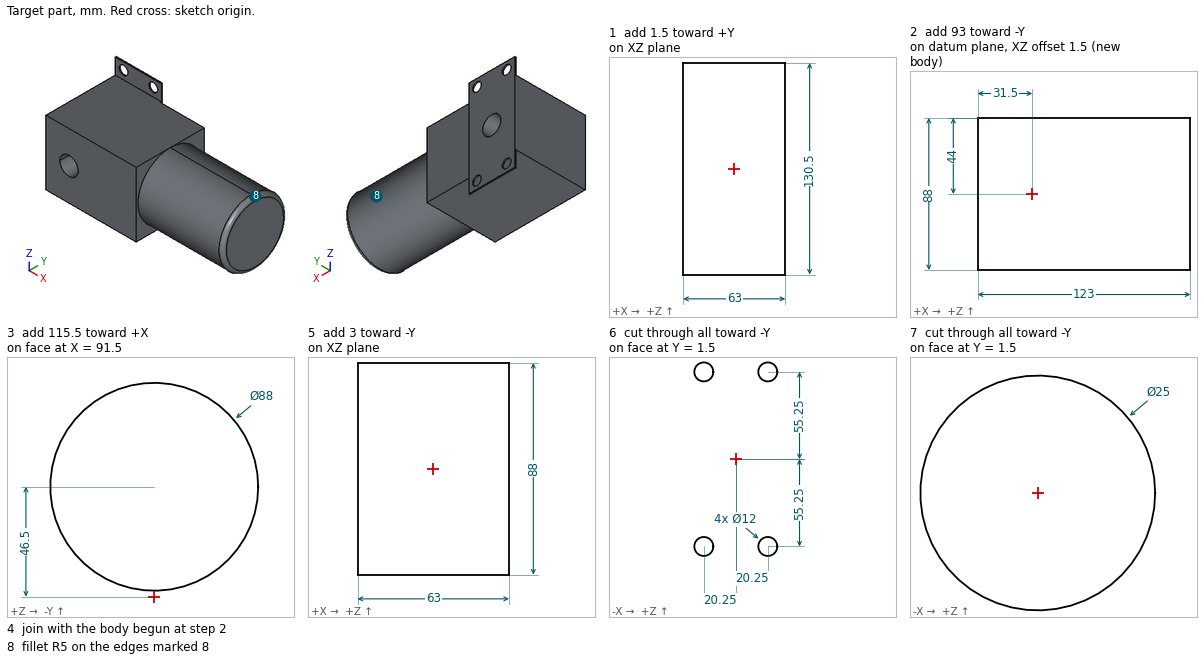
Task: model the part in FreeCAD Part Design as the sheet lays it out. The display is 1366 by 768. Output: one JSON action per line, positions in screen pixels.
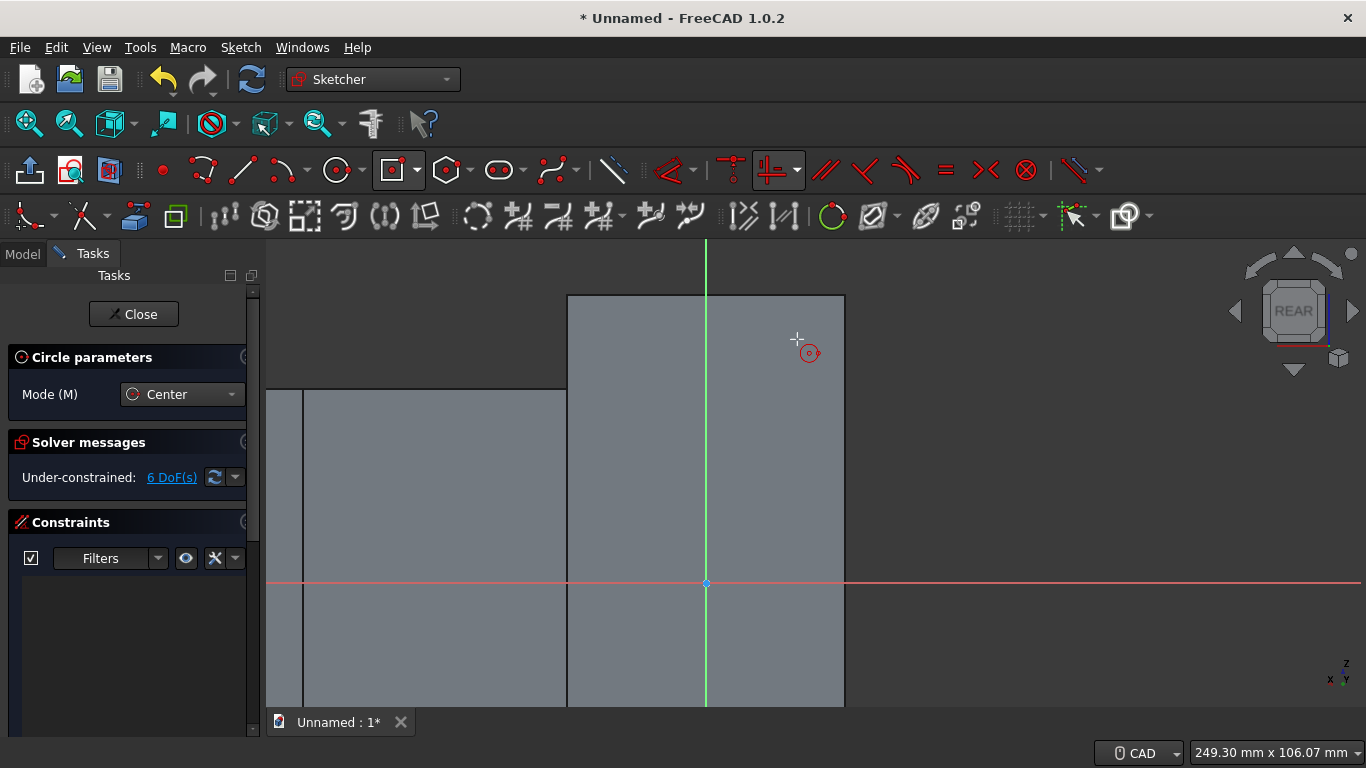
{"action": "left_click", "coordinate": [796, 340]}
{"action": "left_click", "coordinate": [814, 321]}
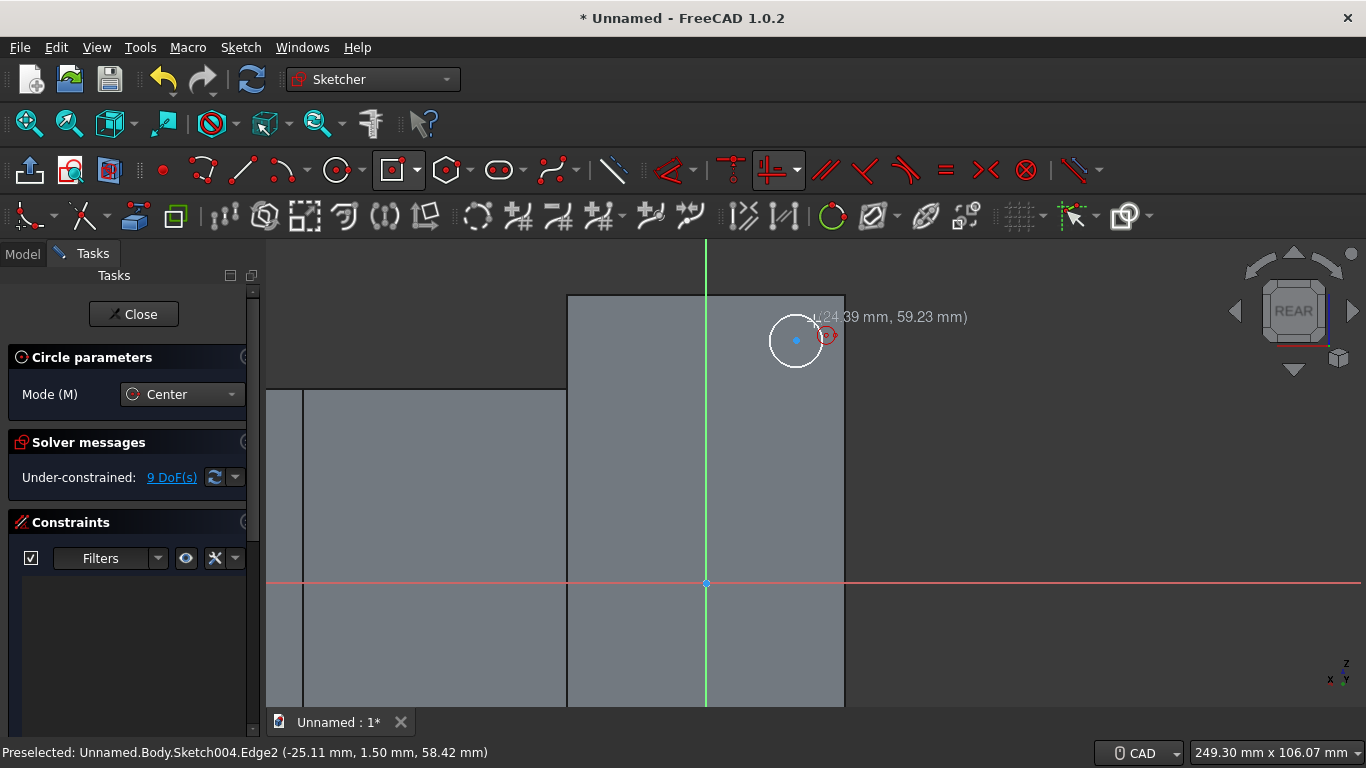
{"action": "left_click", "coordinate": [617, 340]}
{"action": "left_click", "coordinate": [636, 321]}
{"action": "key", "text": "Escape"}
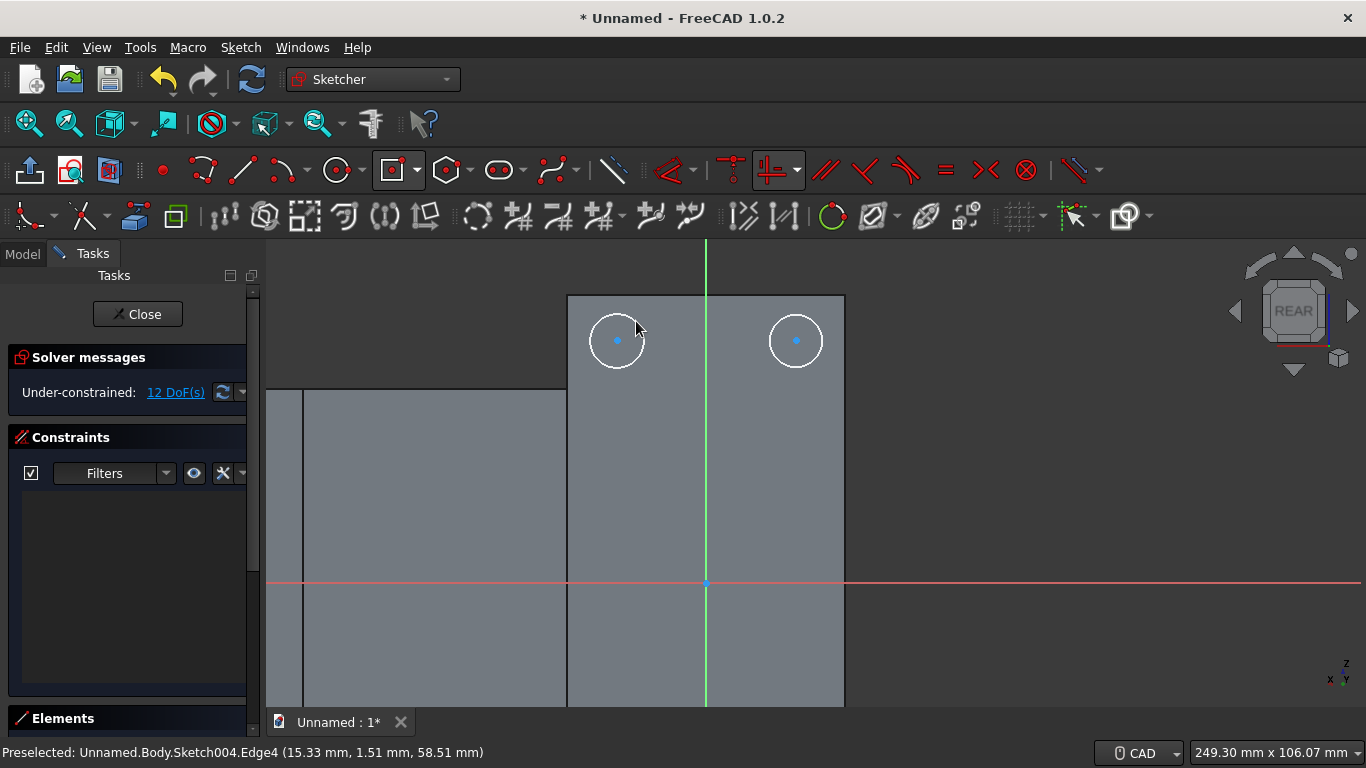
{"action": "scroll", "coordinate": [797, 339], "scroll_direction": "down", "scroll_amount": 3}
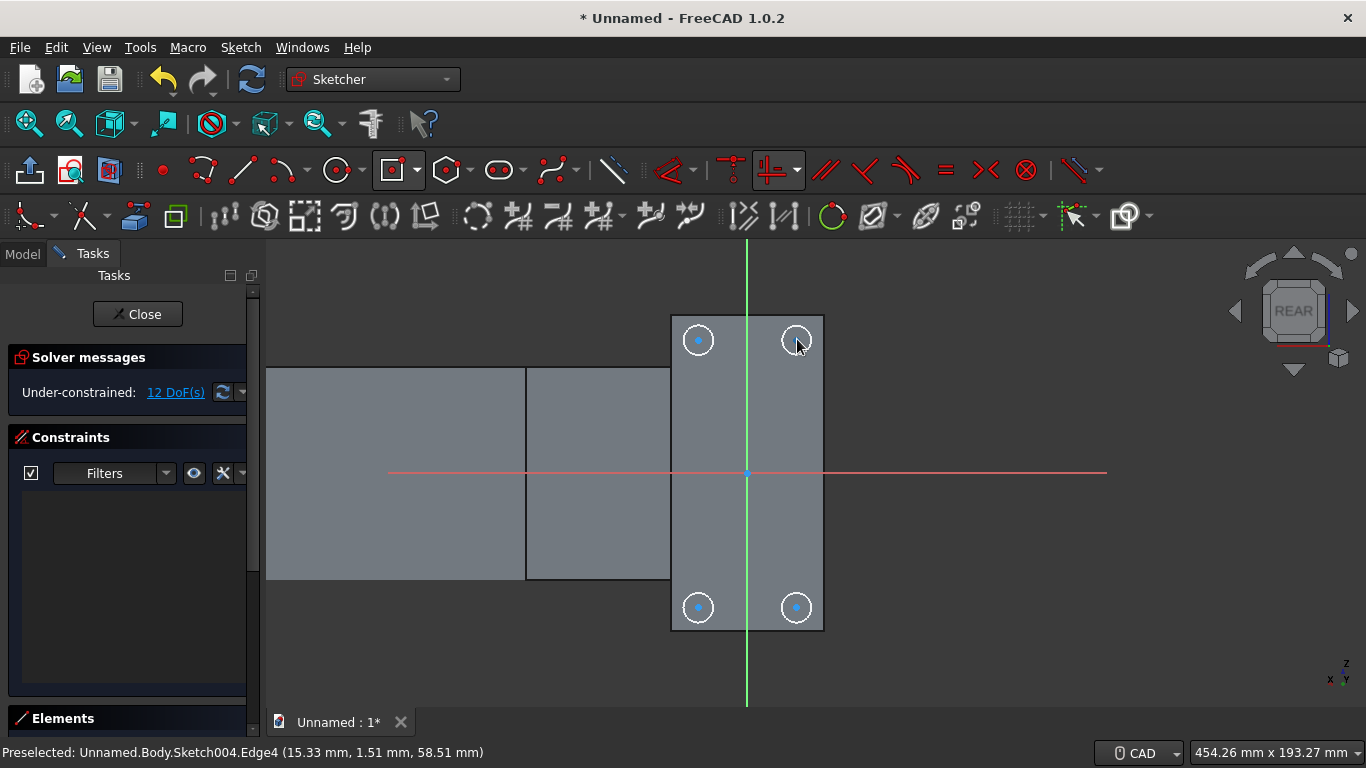
{"action": "left_click", "coordinate": [807, 597]}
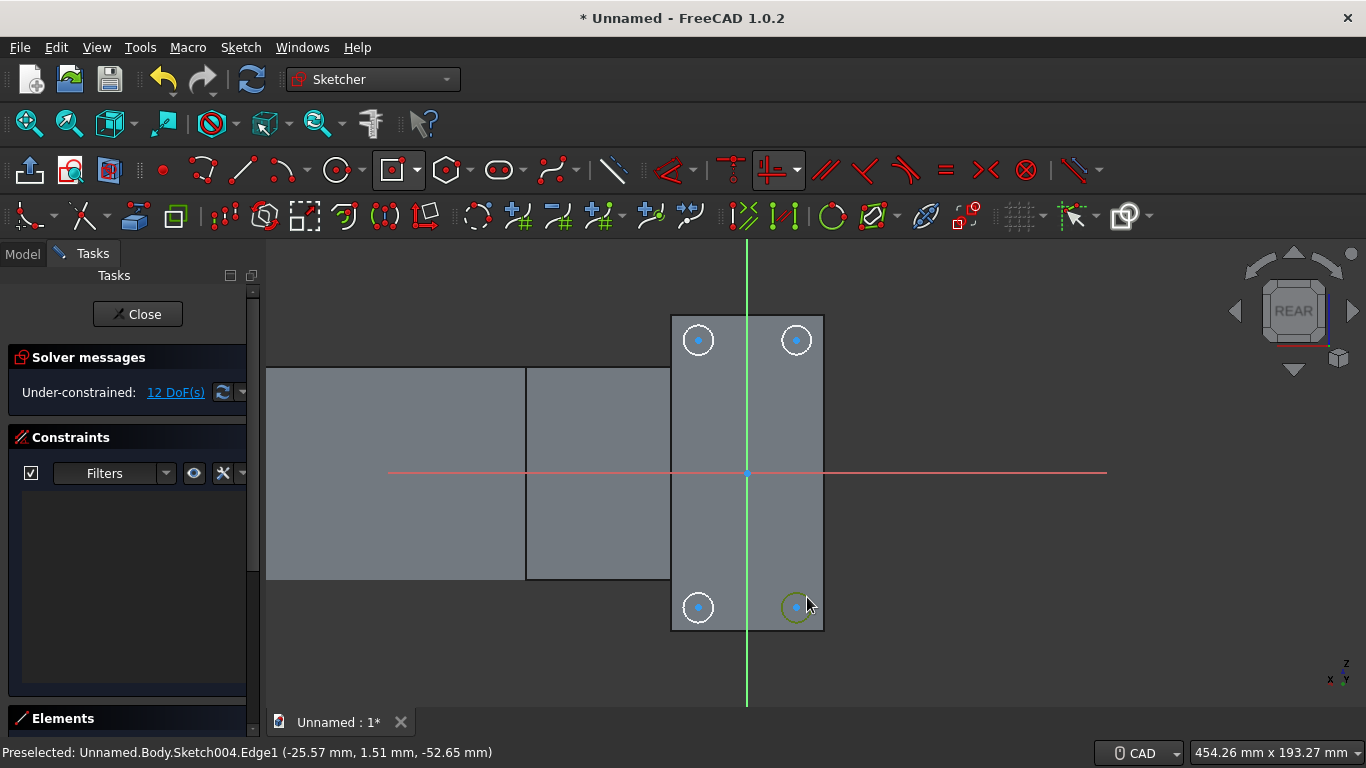
{"action": "left_click", "coordinate": [709, 597]}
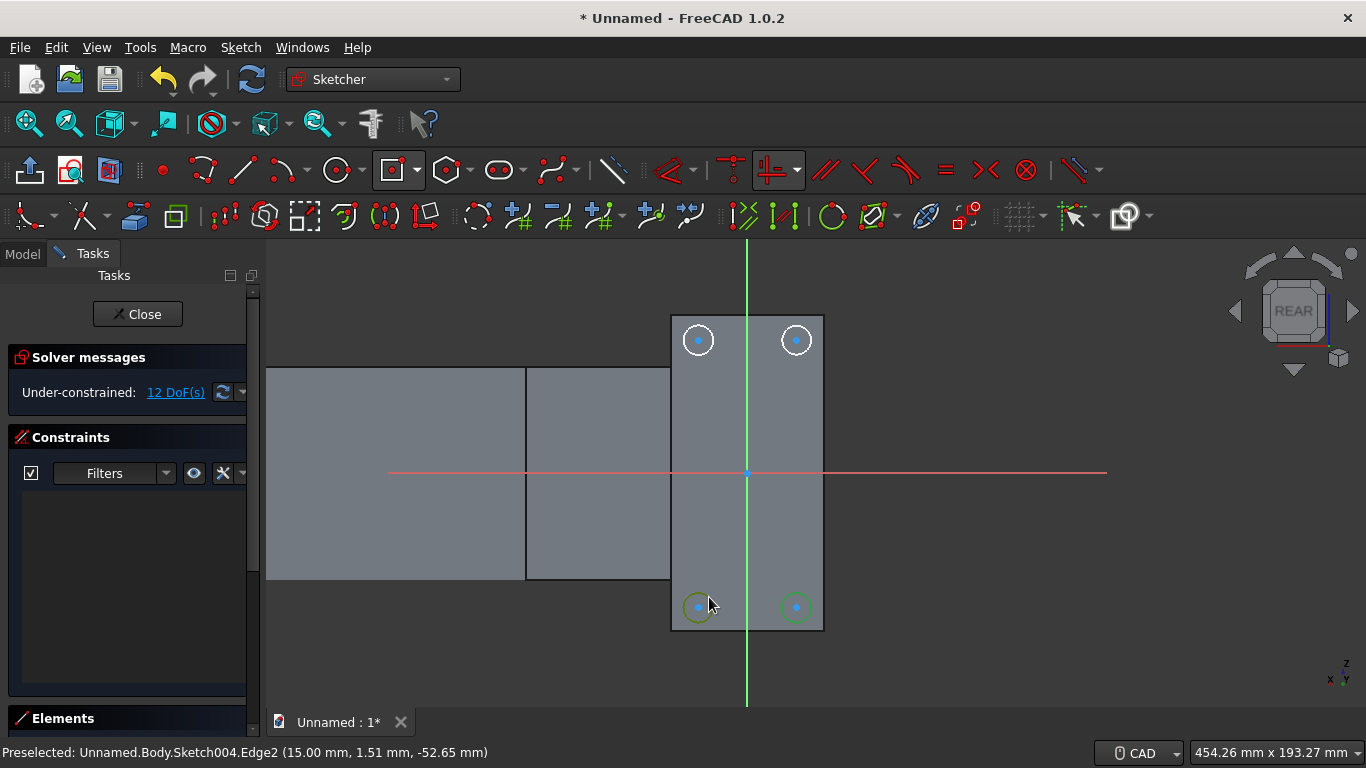
{"action": "left_click", "coordinate": [807, 330]}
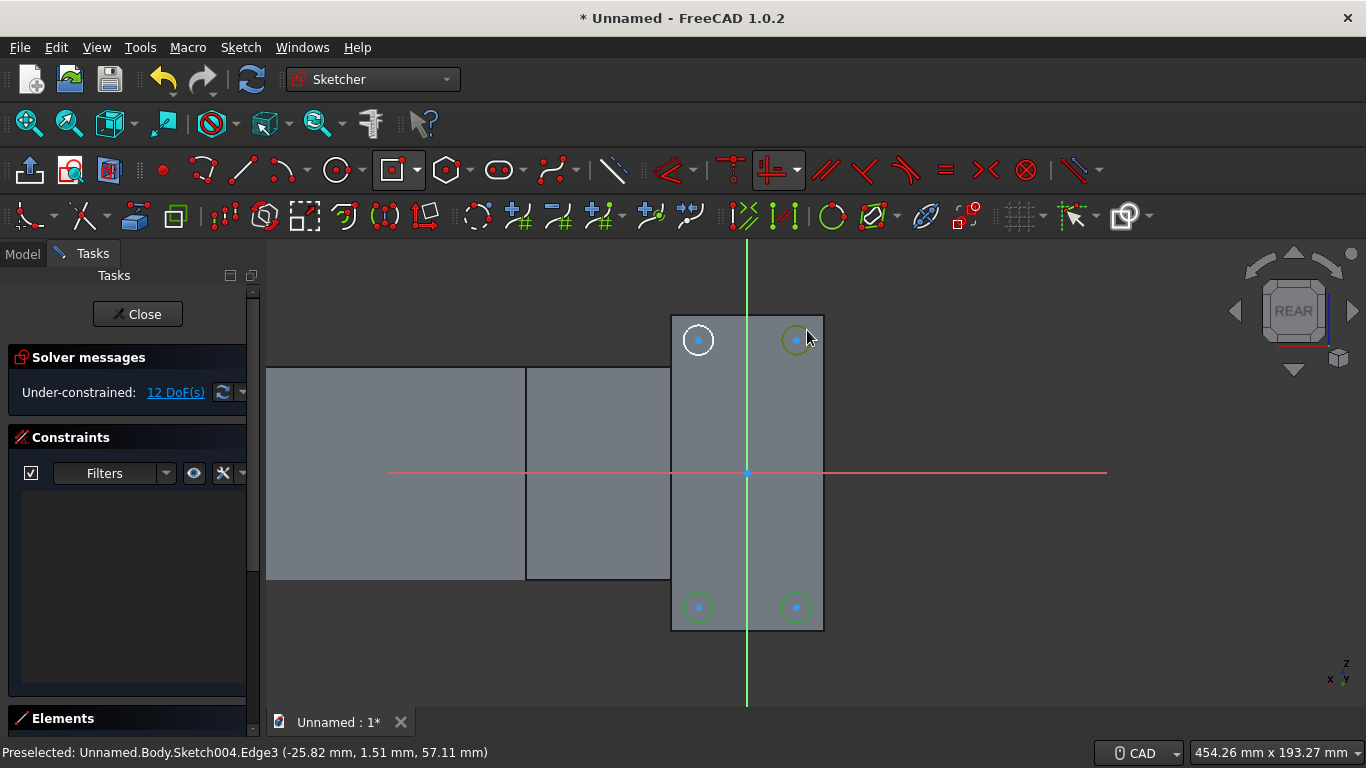
{"action": "left_click", "coordinate": [709, 330]}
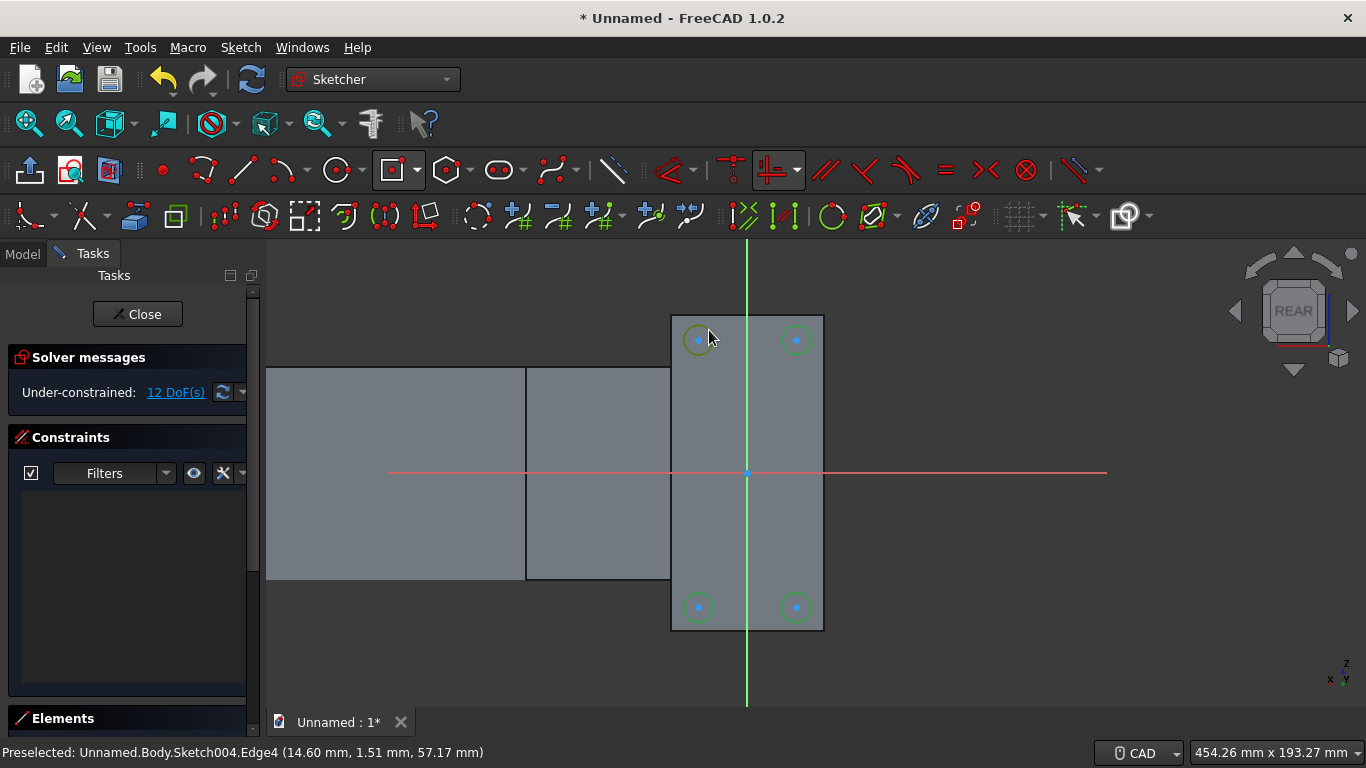
{"action": "left_click", "coordinate": [946, 170]}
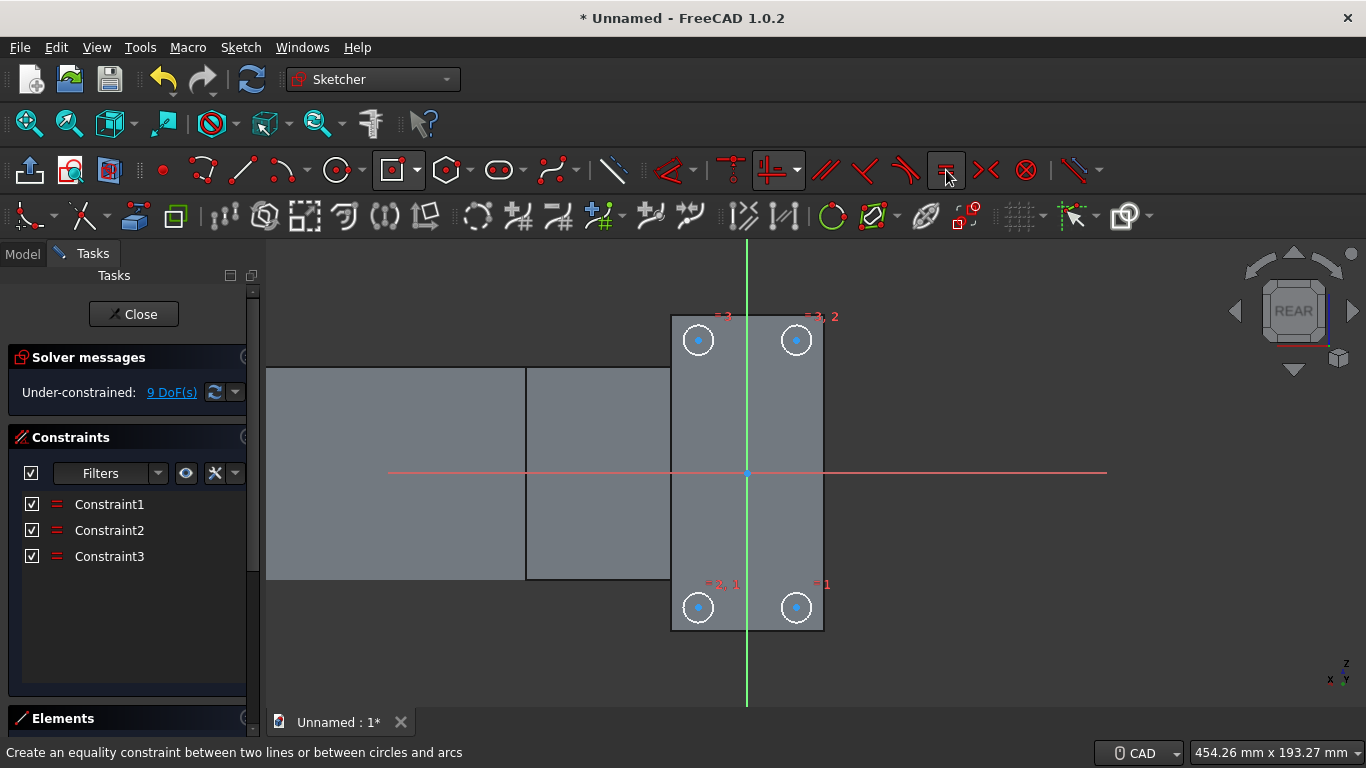
{"action": "left_click", "coordinate": [796, 608]}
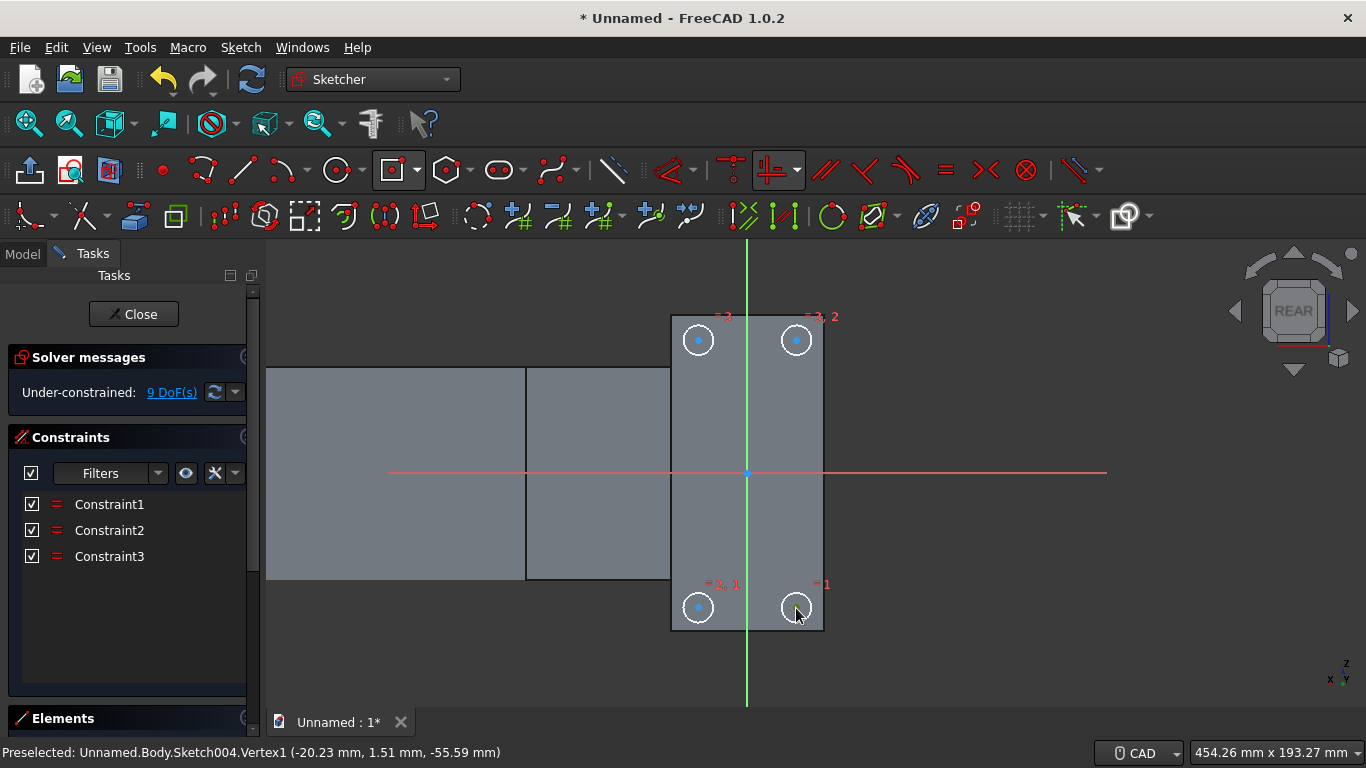
{"action": "left_click", "coordinate": [698, 608]}